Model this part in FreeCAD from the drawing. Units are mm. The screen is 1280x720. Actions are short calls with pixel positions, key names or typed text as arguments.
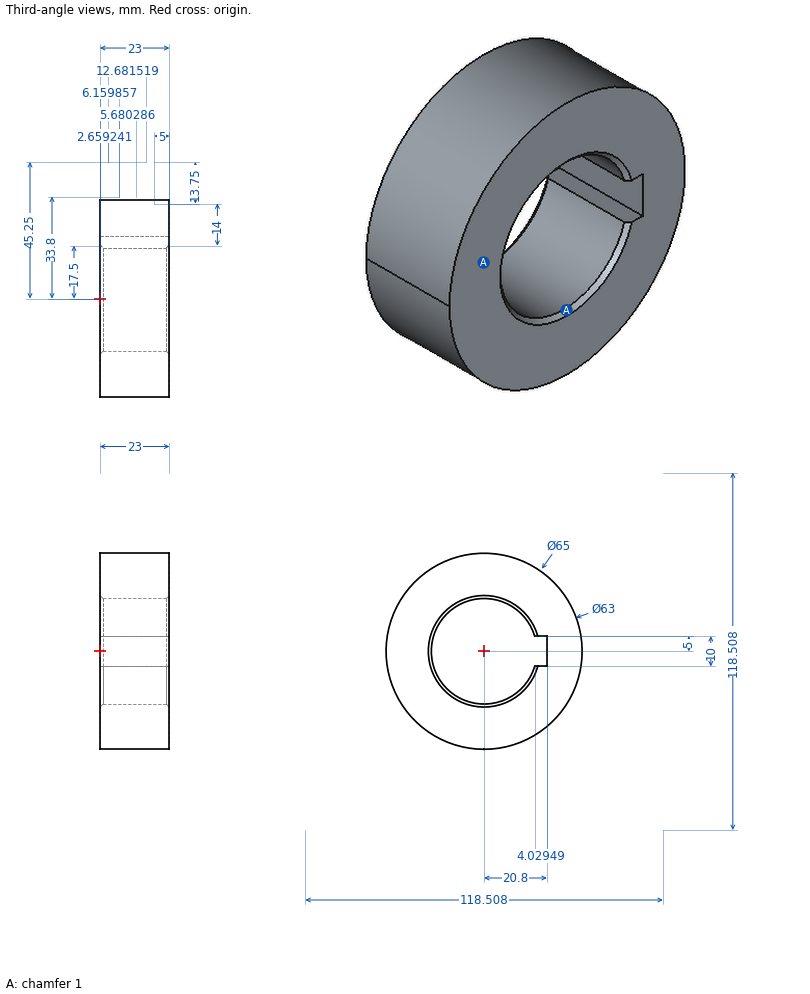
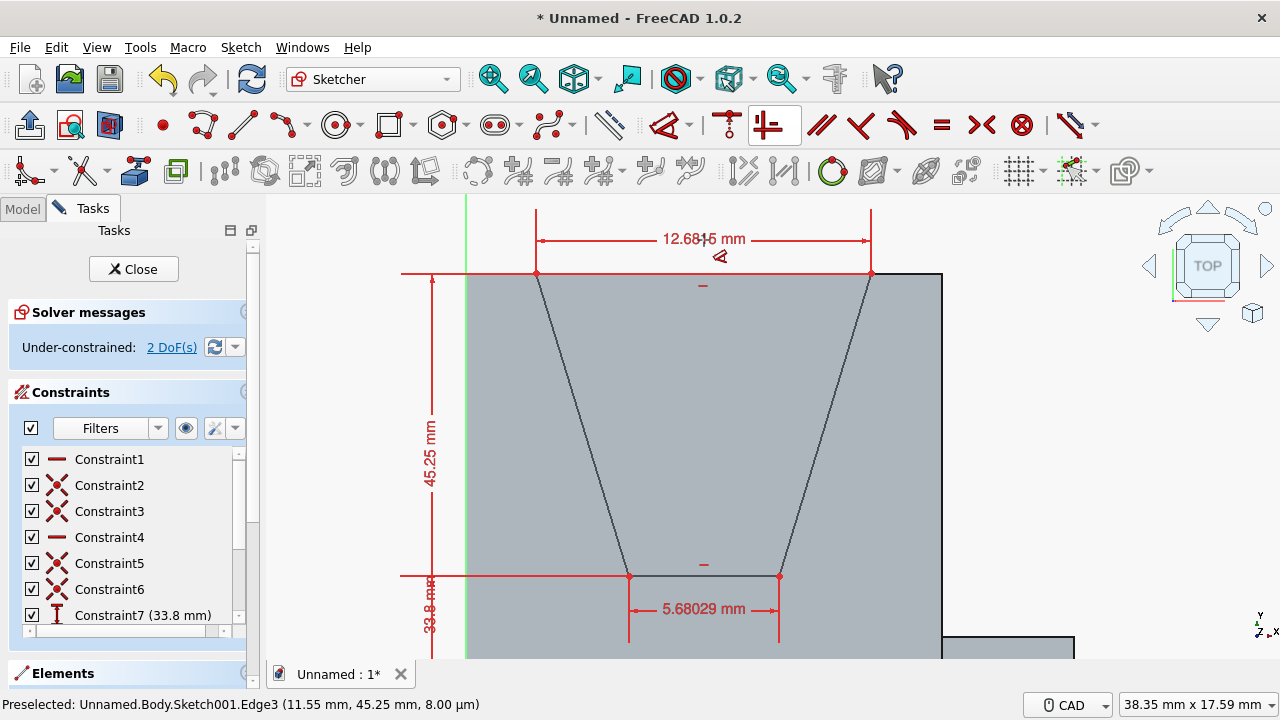
click(629, 576)
click(547, 542)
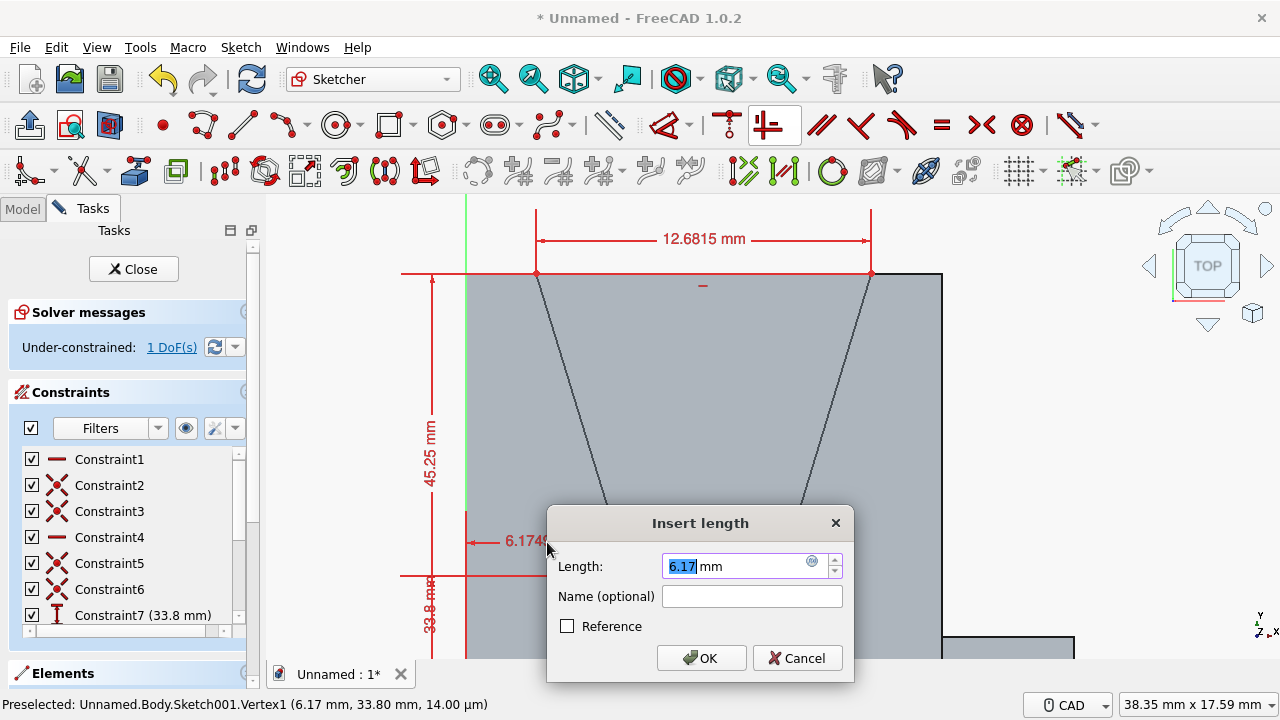
text(6.159857)
key(Return)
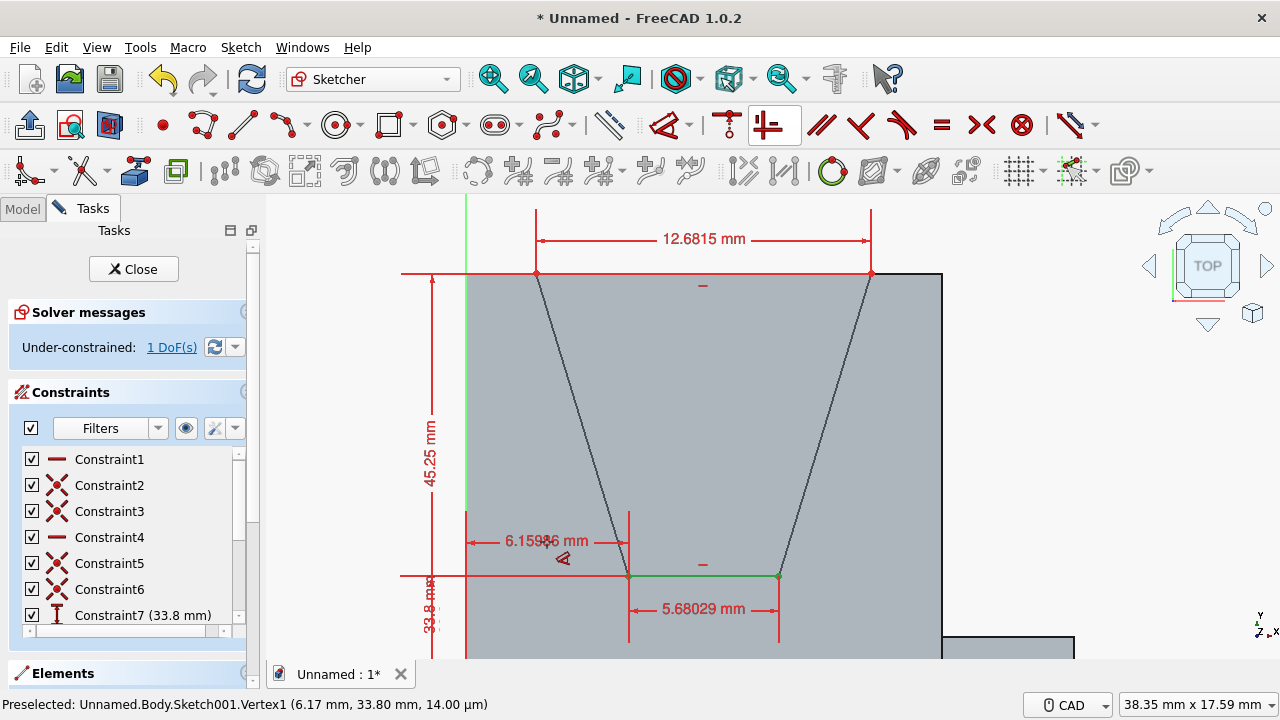
click(536, 274)
click(501, 240)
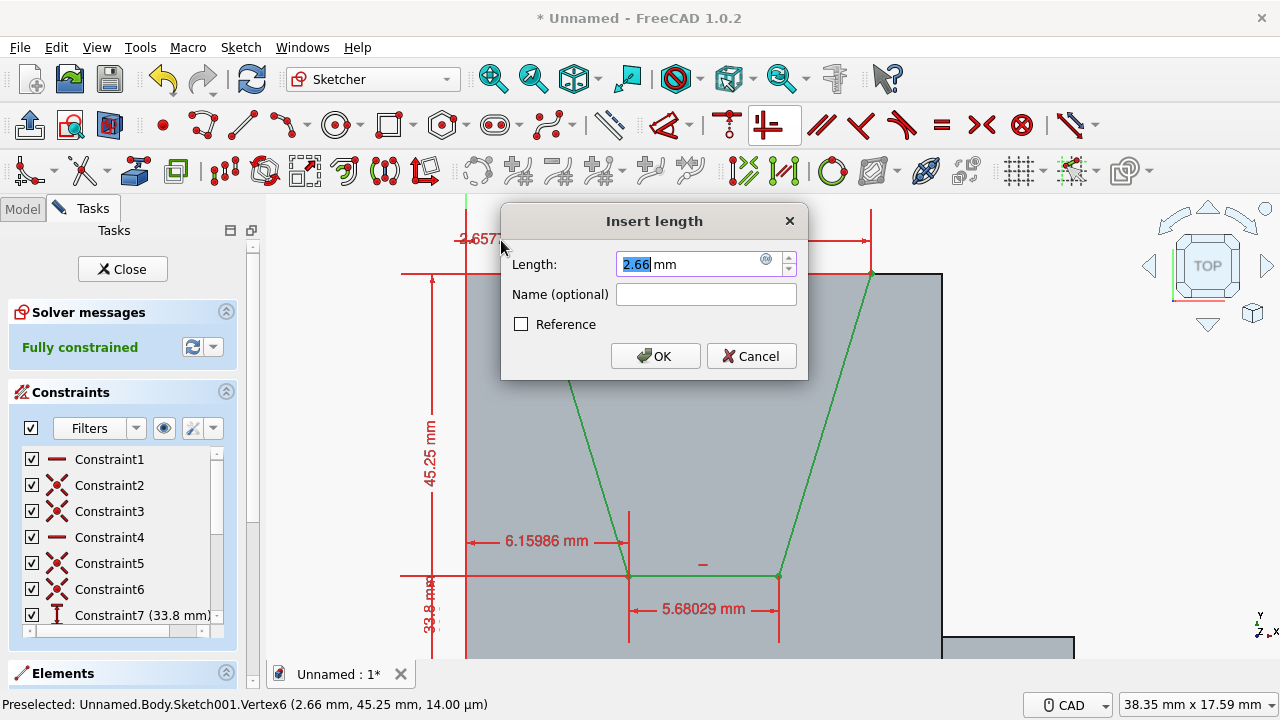
text(2.659241)
key(Return)
key(Escape)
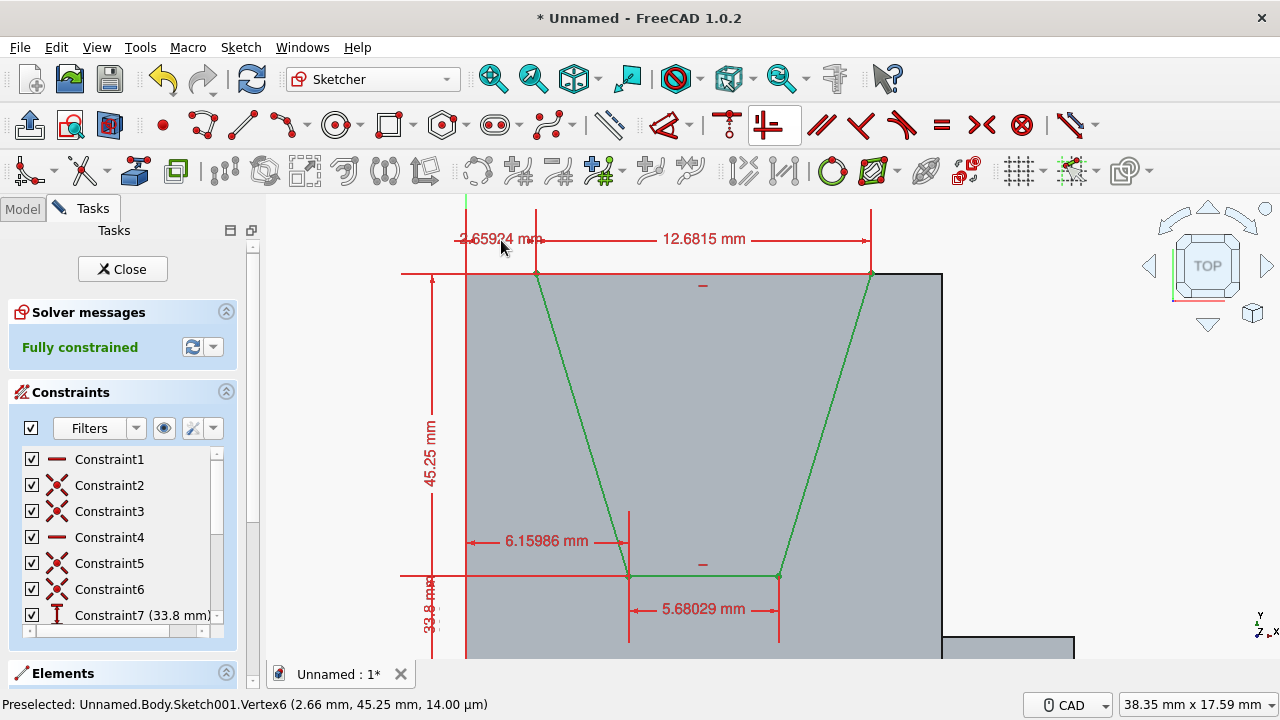
click(123, 269)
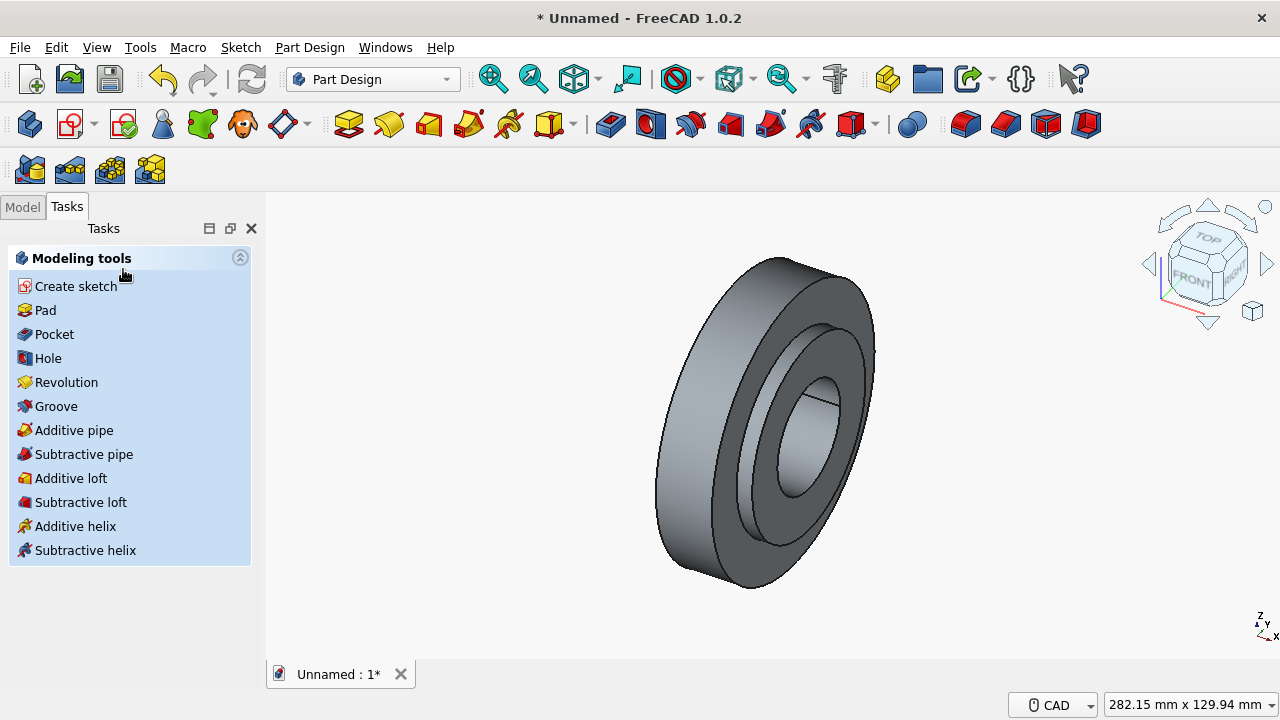
click(692, 124)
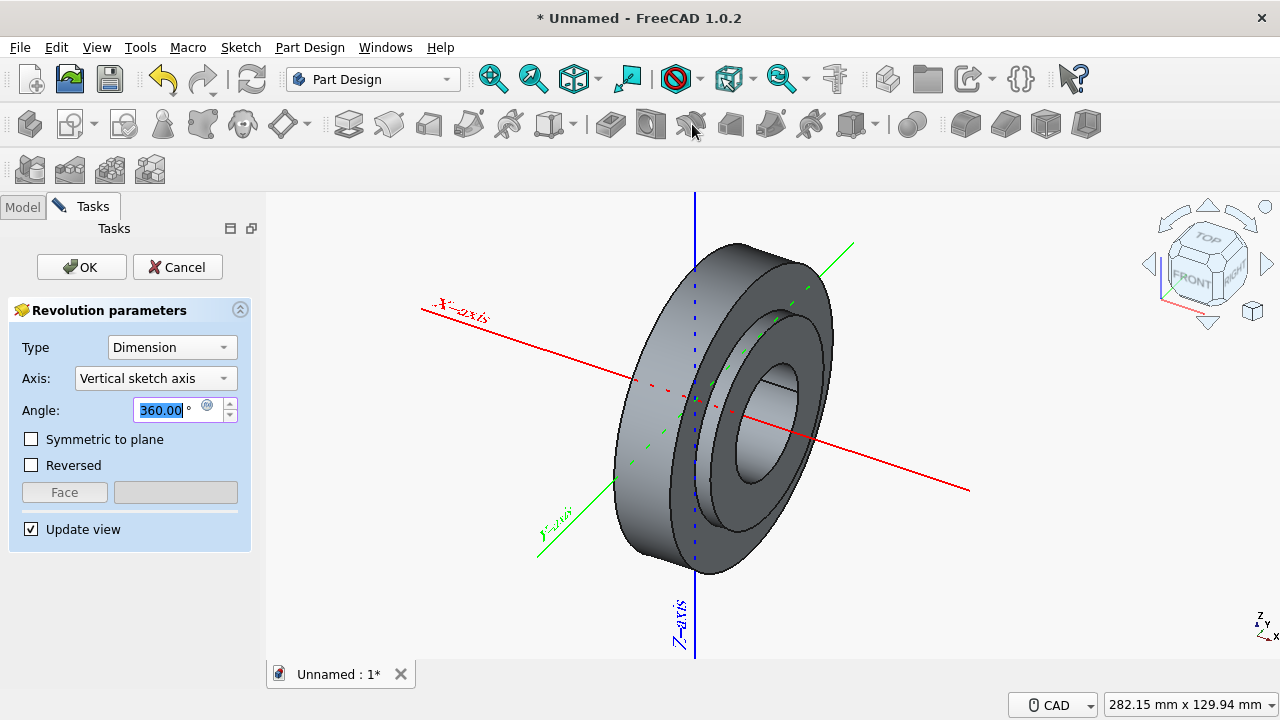
click(156, 378)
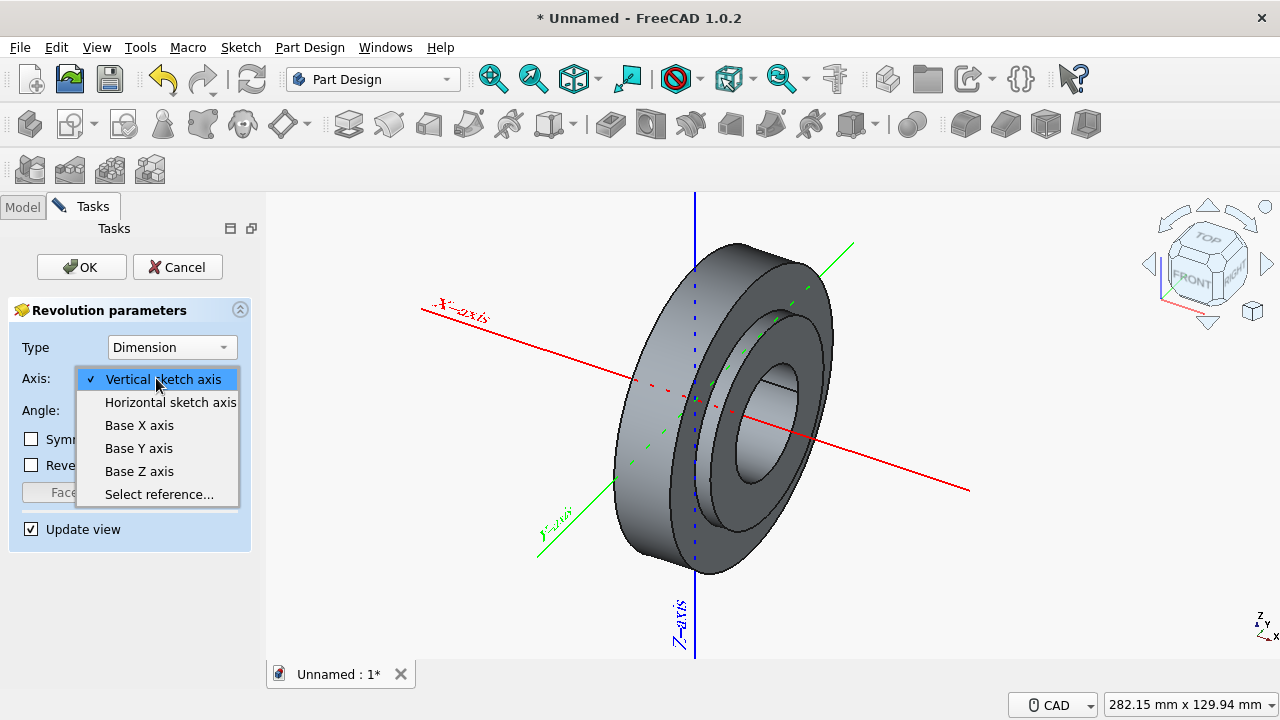
click(156, 402)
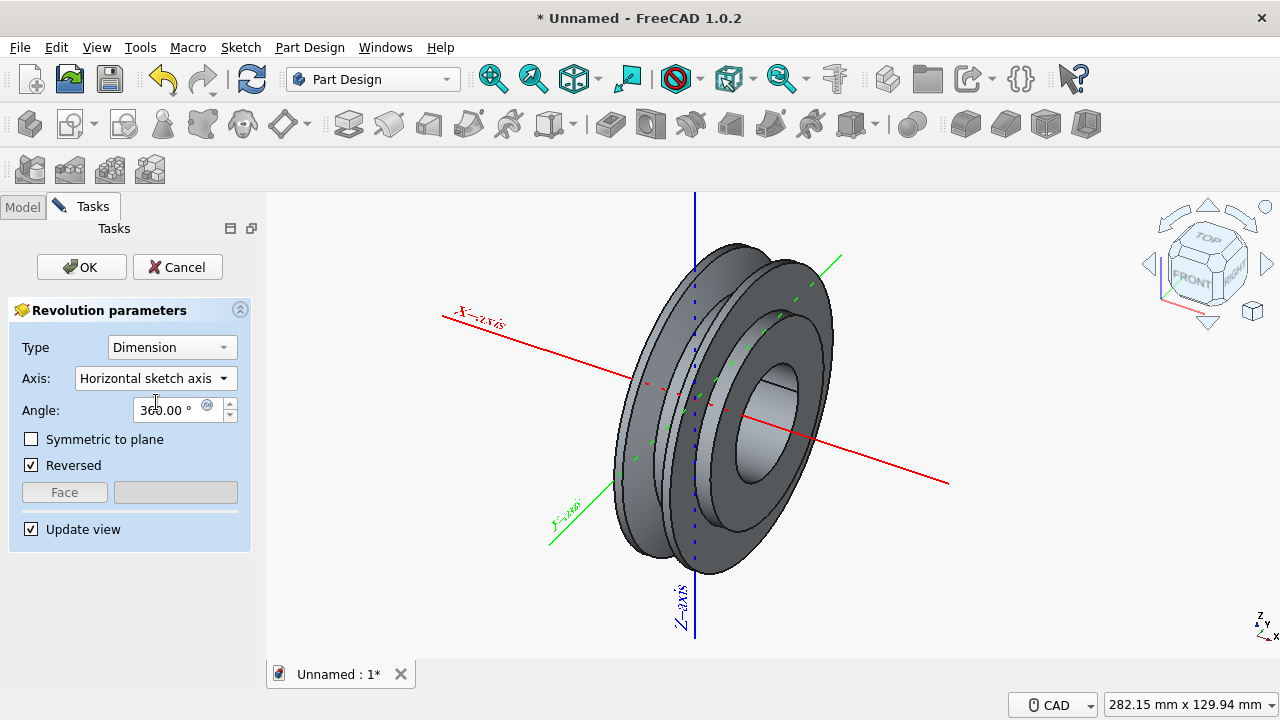
click(82, 267)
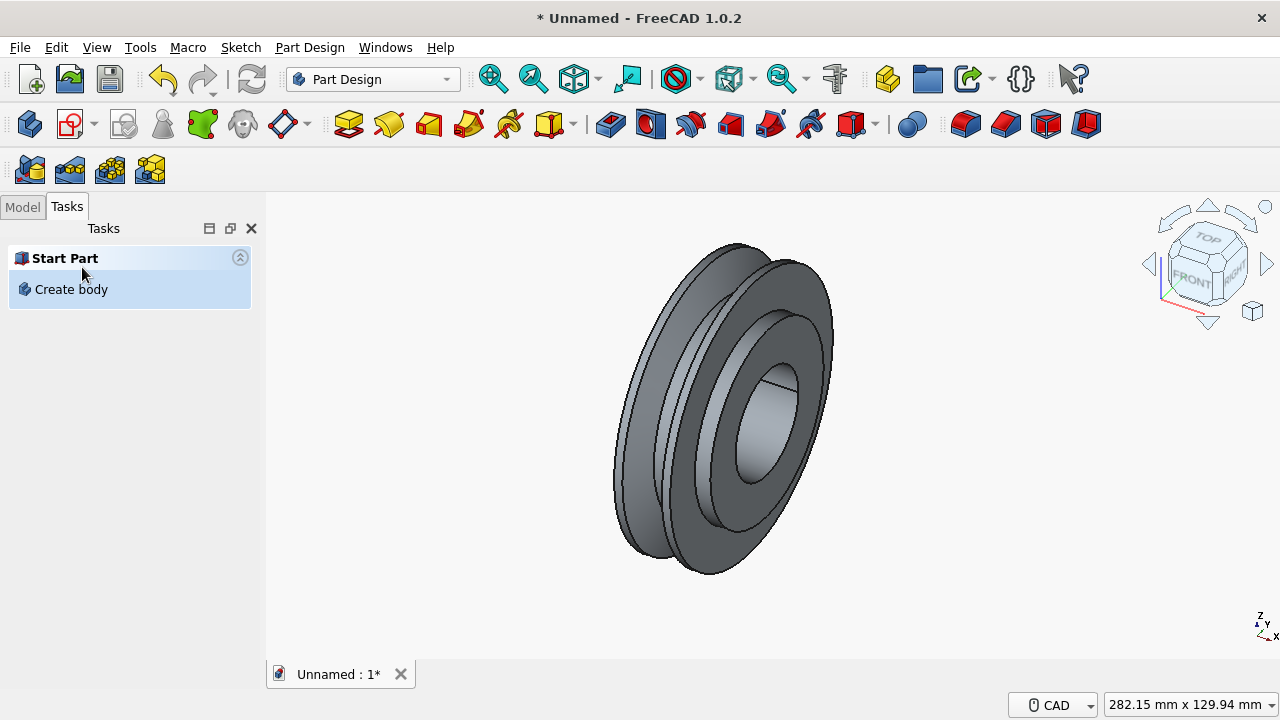
key(v)
key(f)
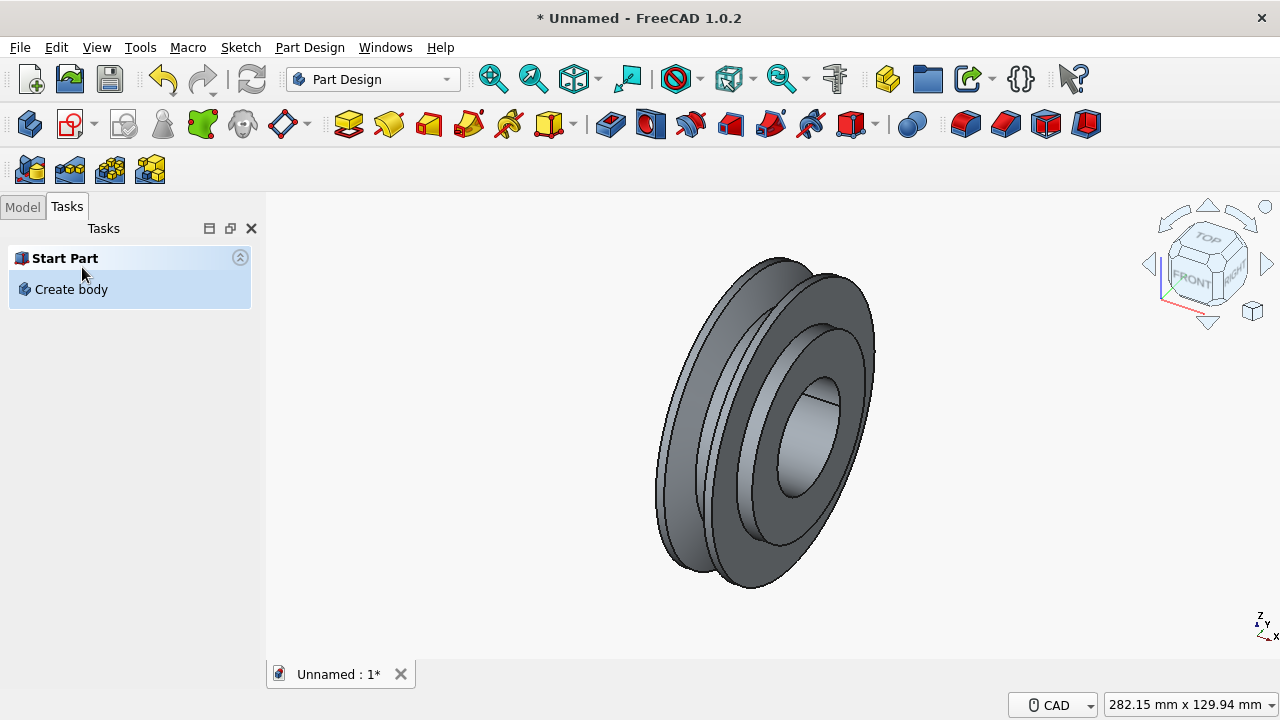
click(799, 495)